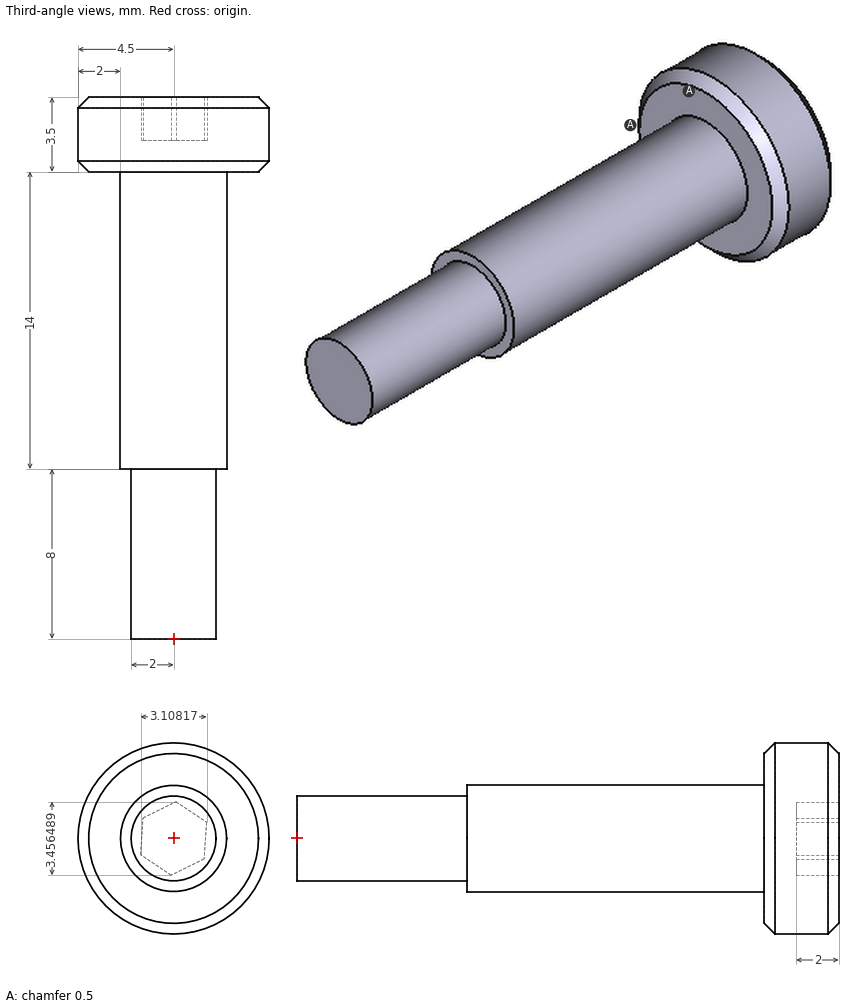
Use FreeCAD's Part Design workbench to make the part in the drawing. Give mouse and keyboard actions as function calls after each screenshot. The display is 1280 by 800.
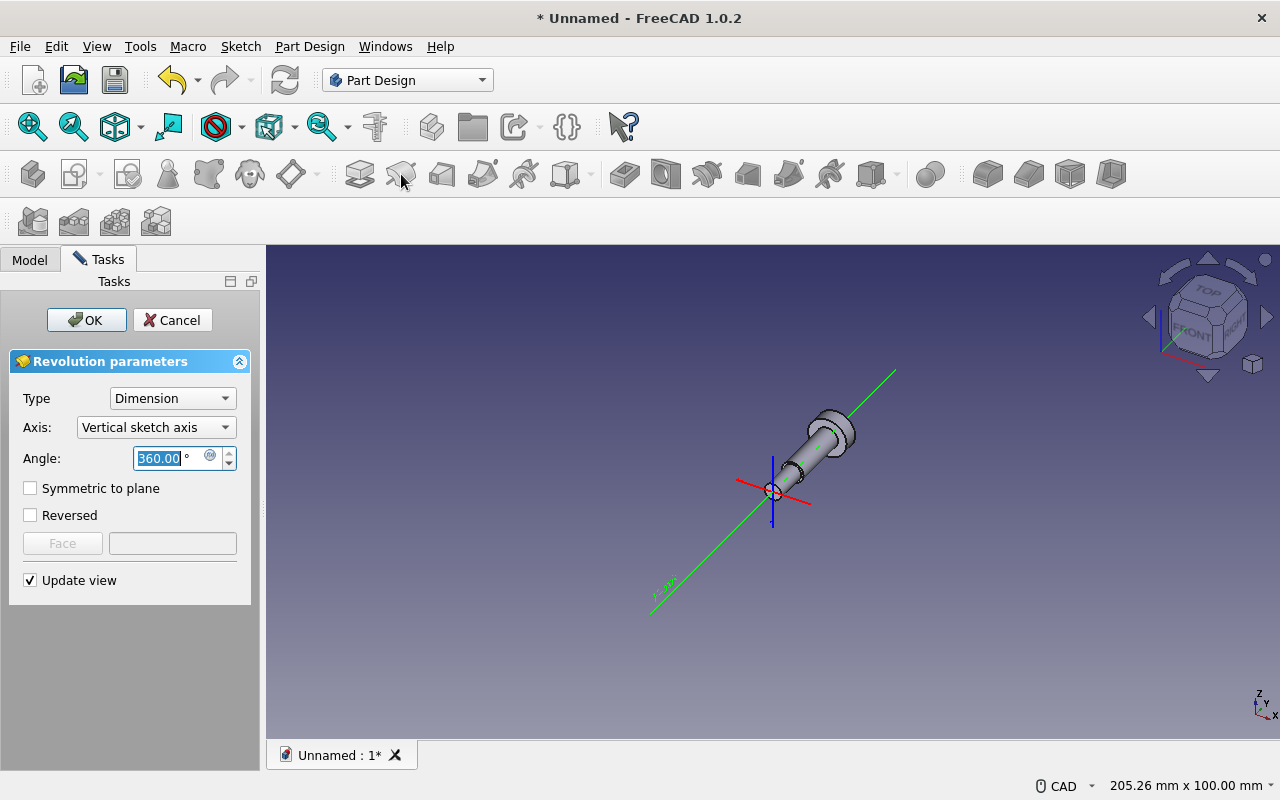
click(87, 320)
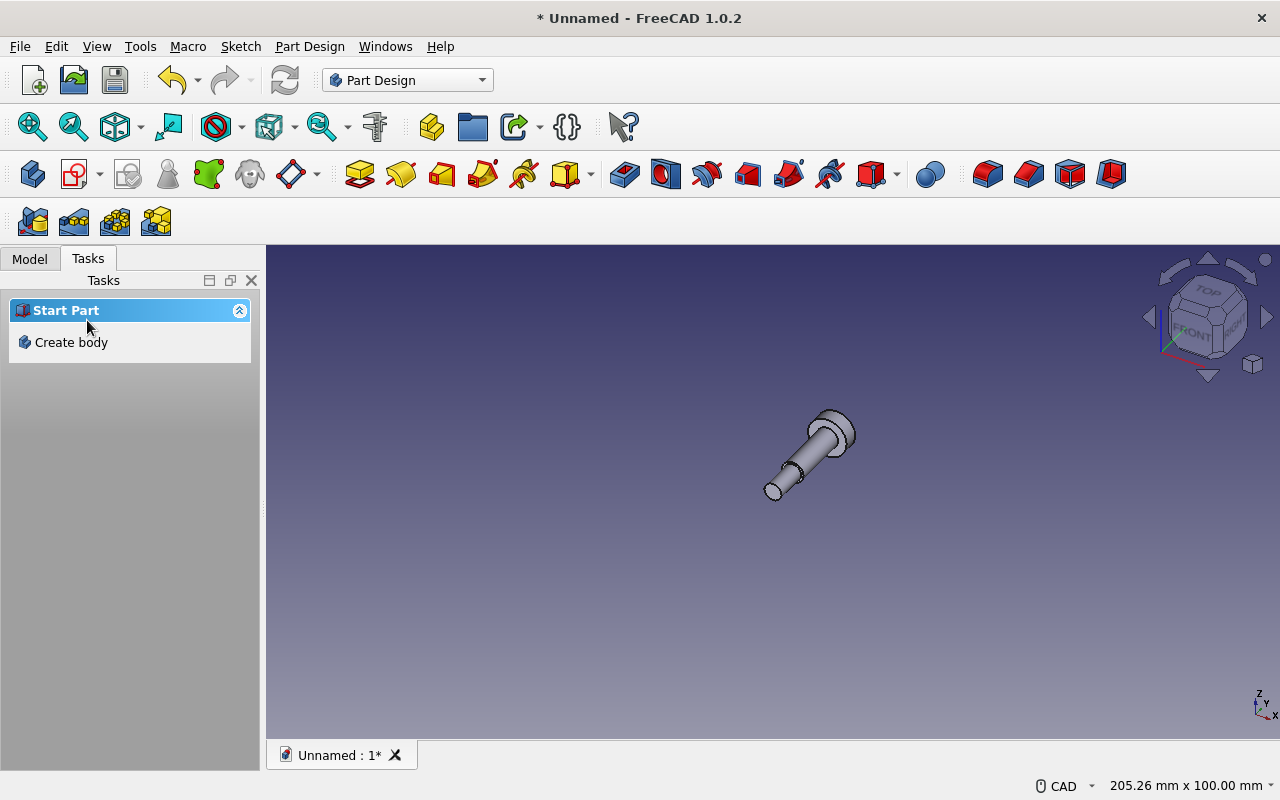
click(33, 128)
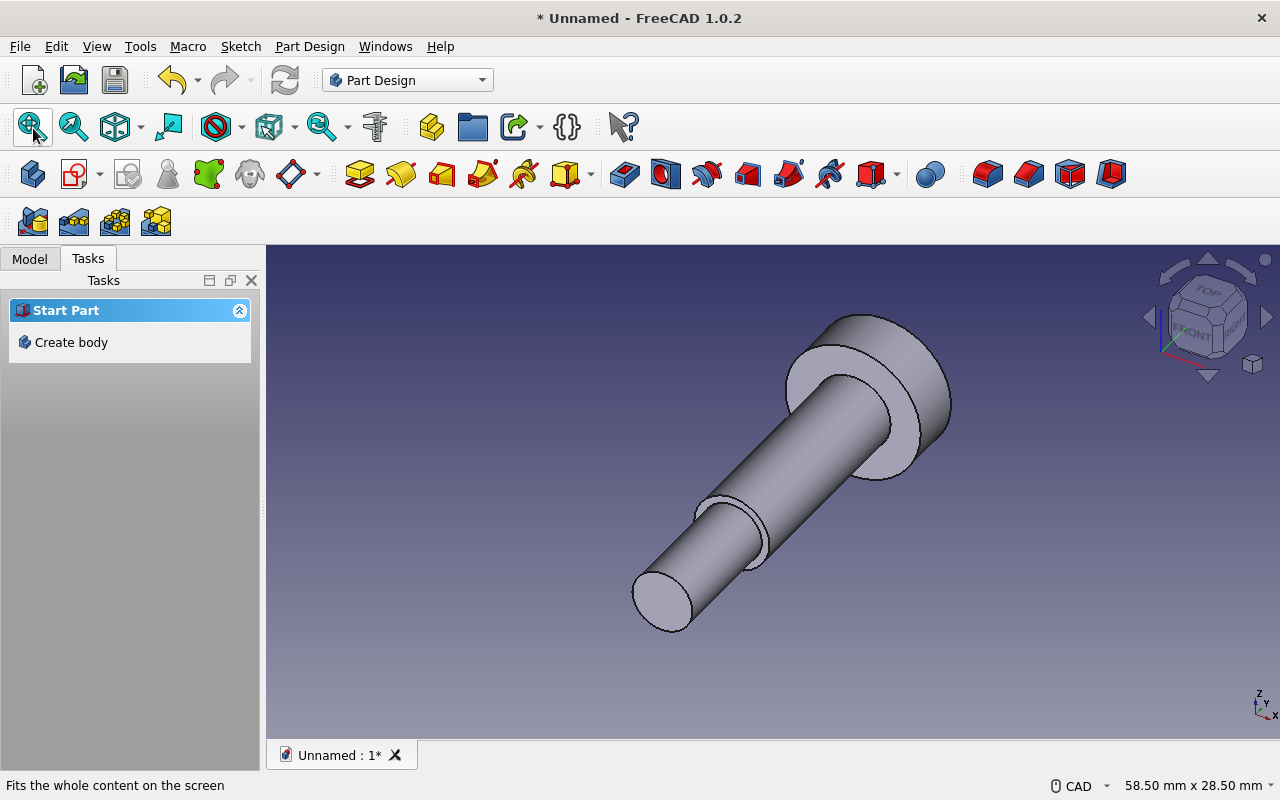
key(4)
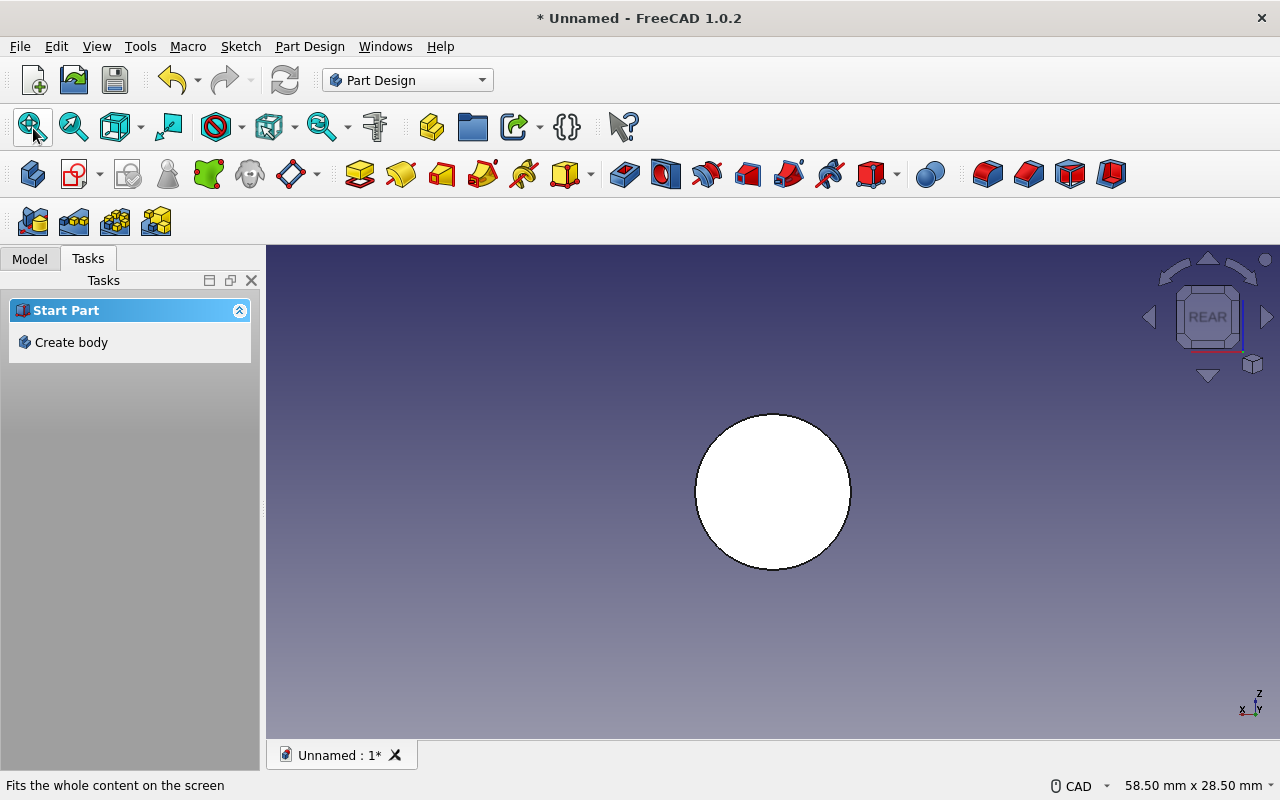
click(33, 128)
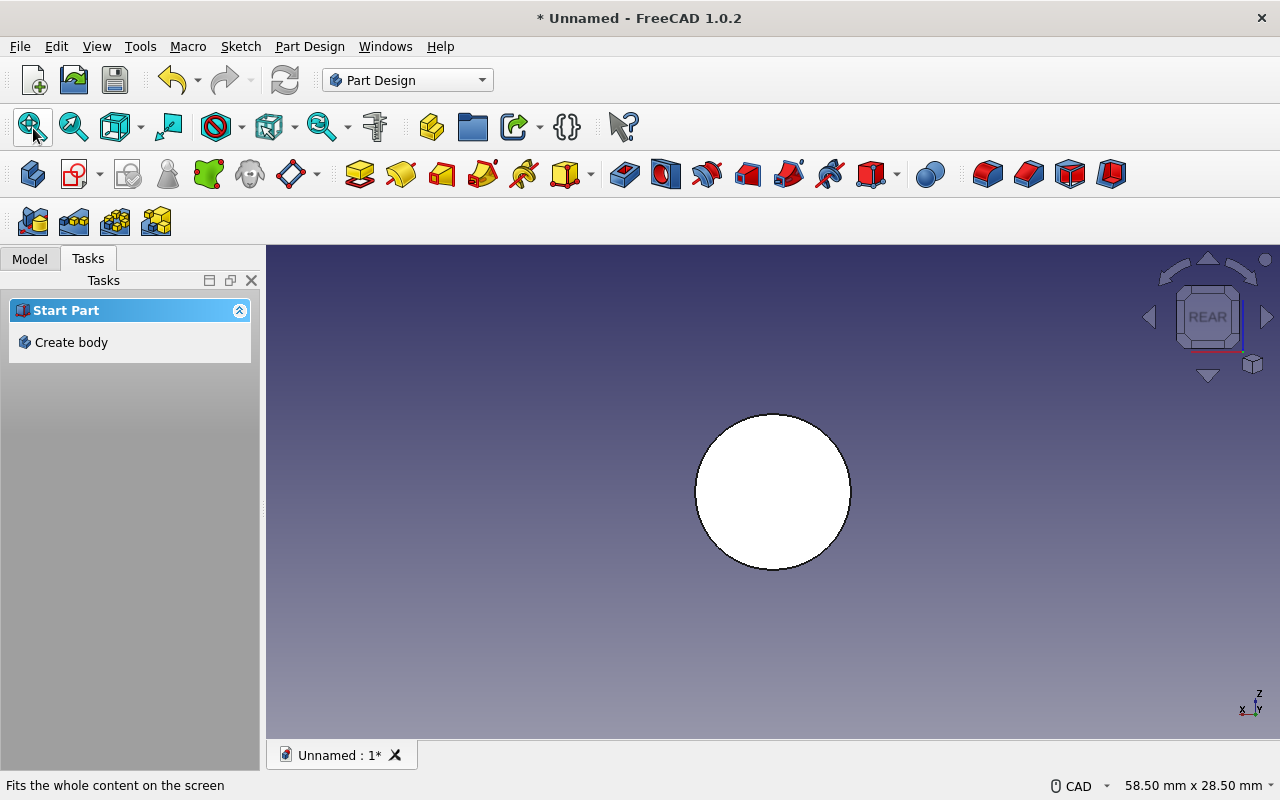
click(773, 491)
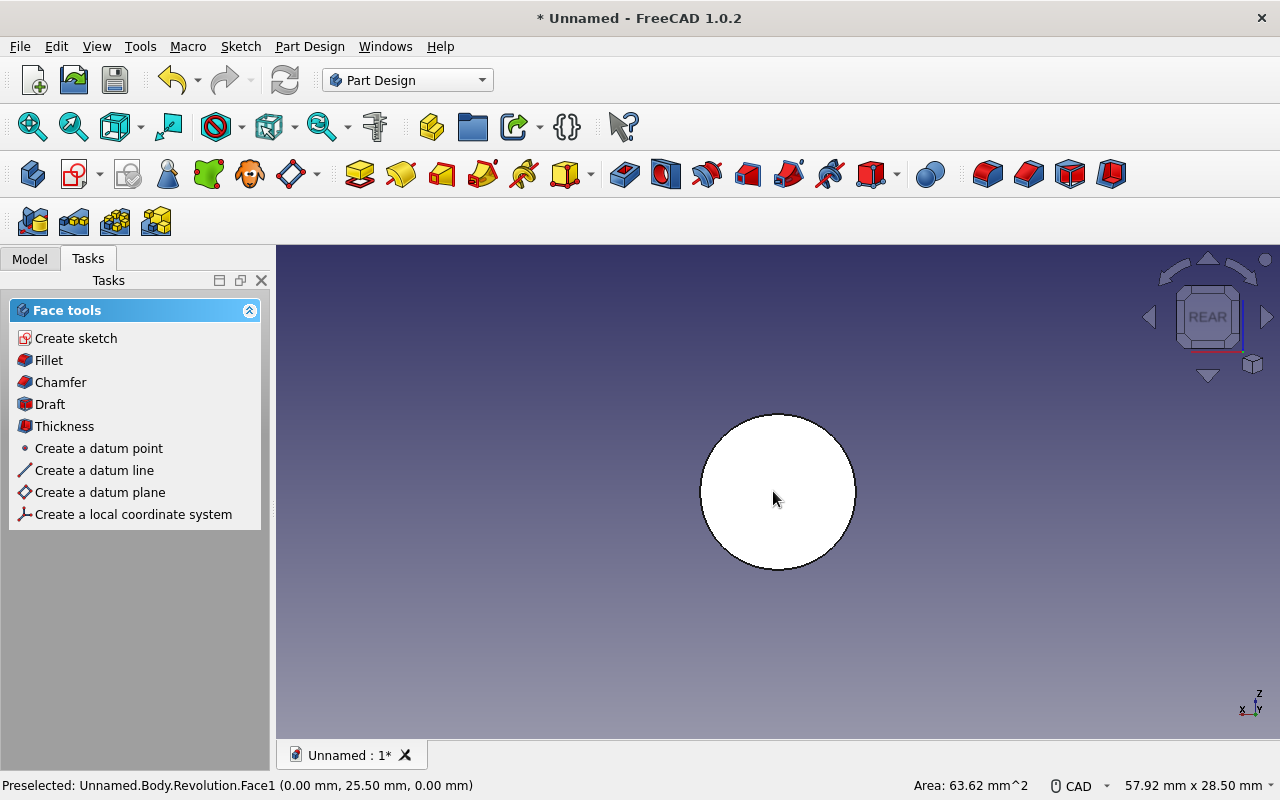
click(74, 174)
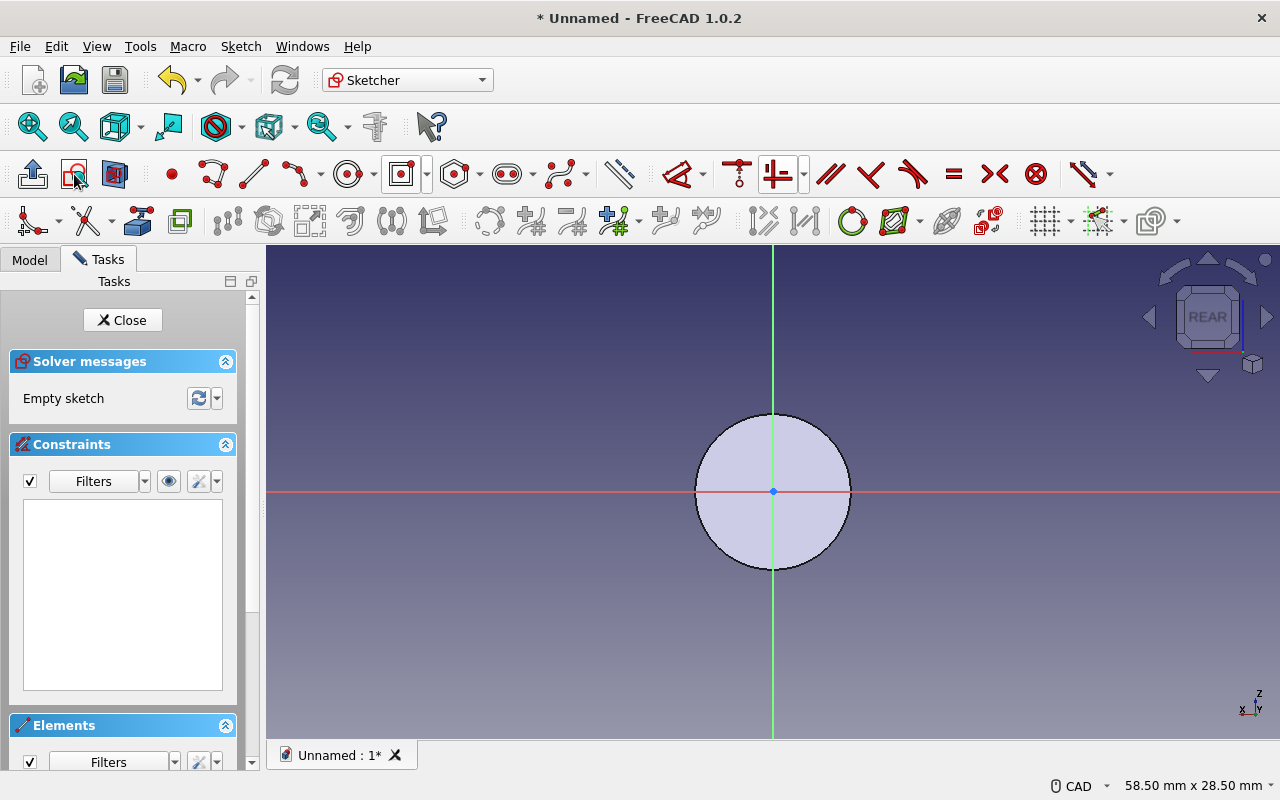
scroll(790, 492, up, 8)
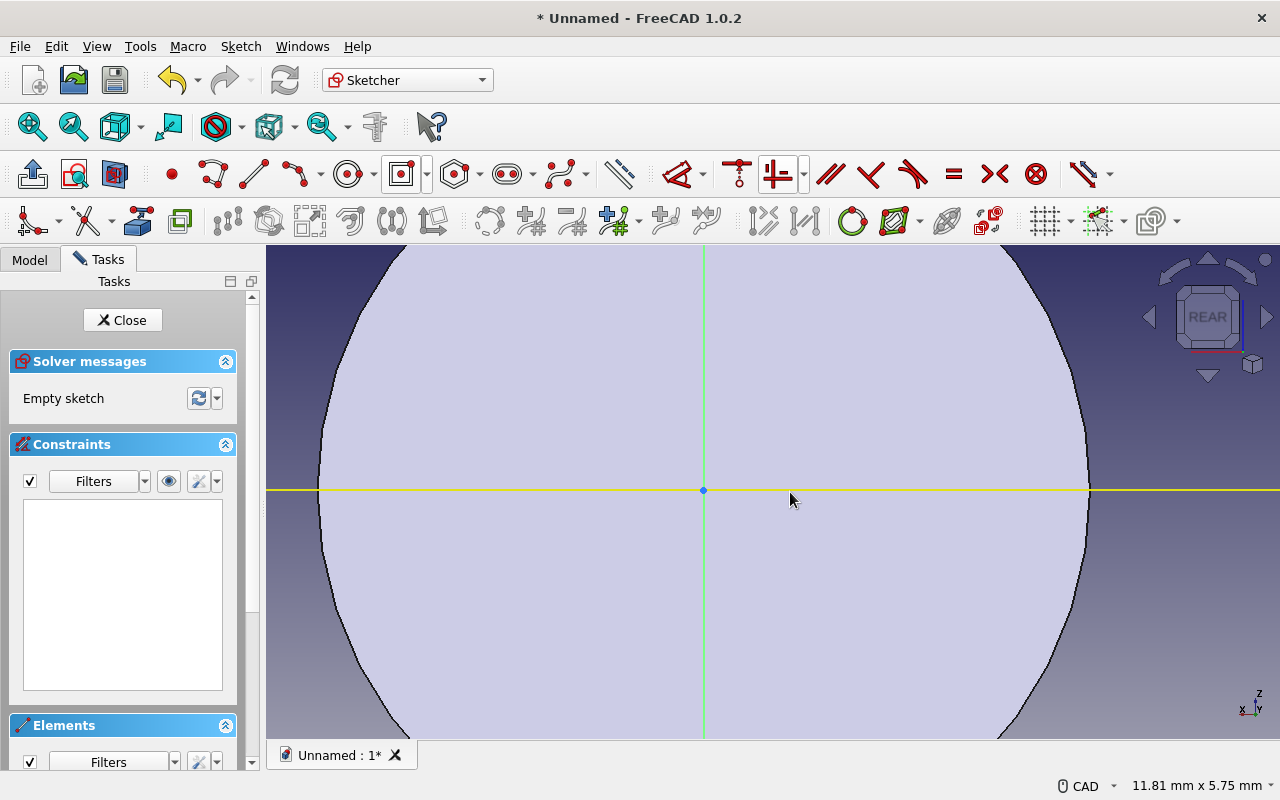
click(454, 174)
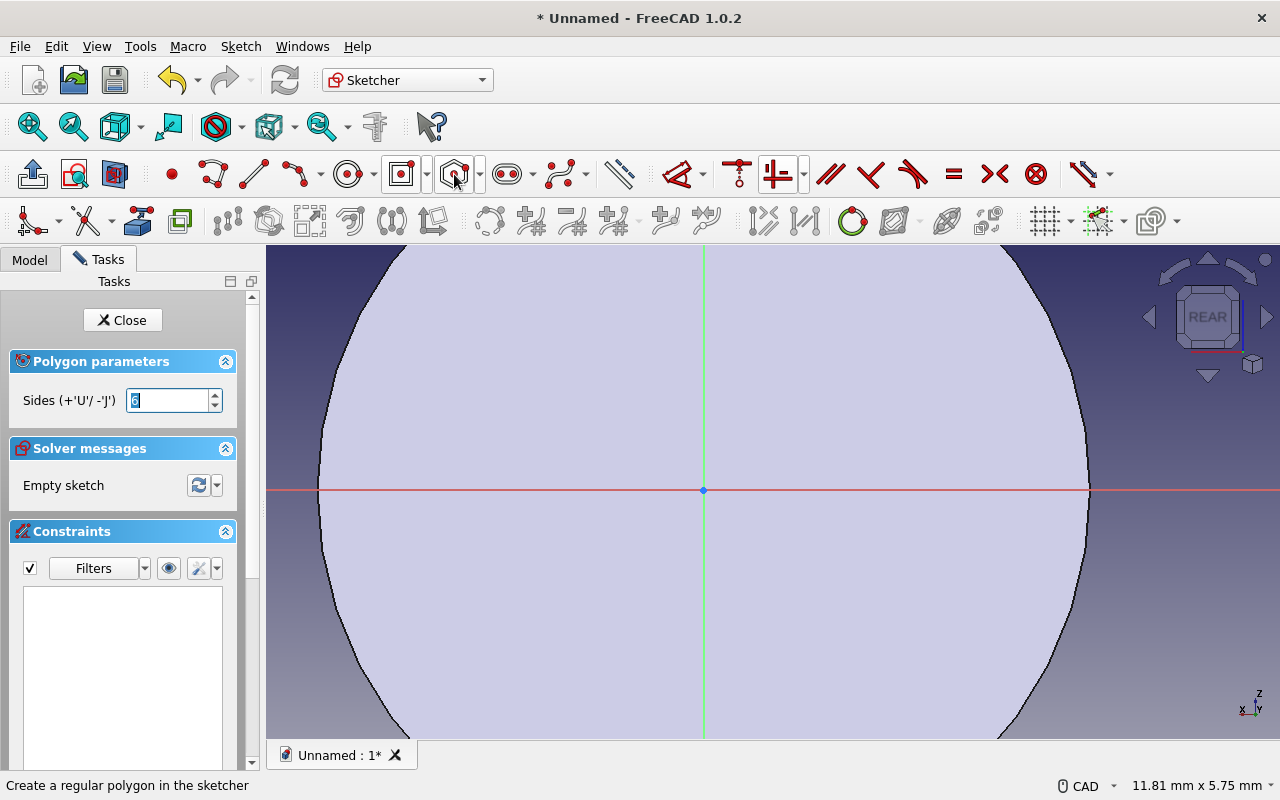
click(704, 490)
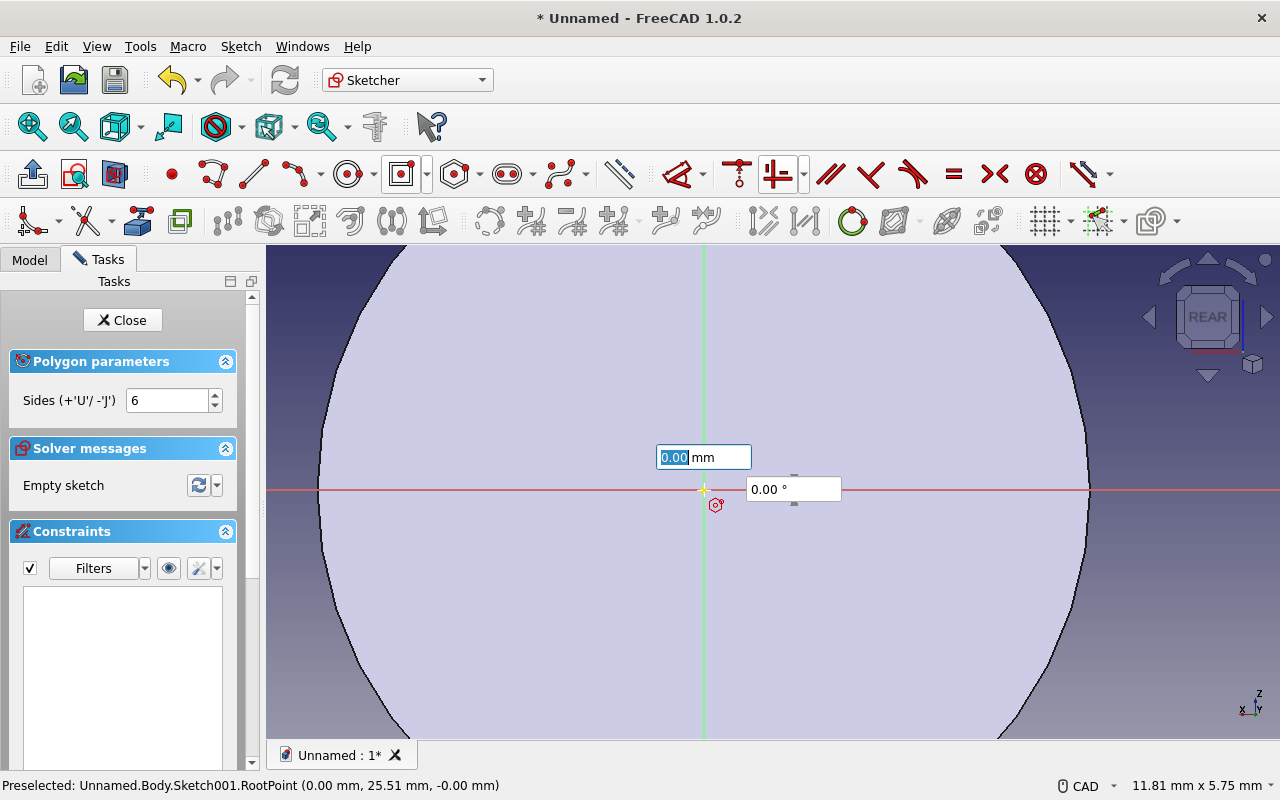
click(580, 573)
right_click(580, 573)